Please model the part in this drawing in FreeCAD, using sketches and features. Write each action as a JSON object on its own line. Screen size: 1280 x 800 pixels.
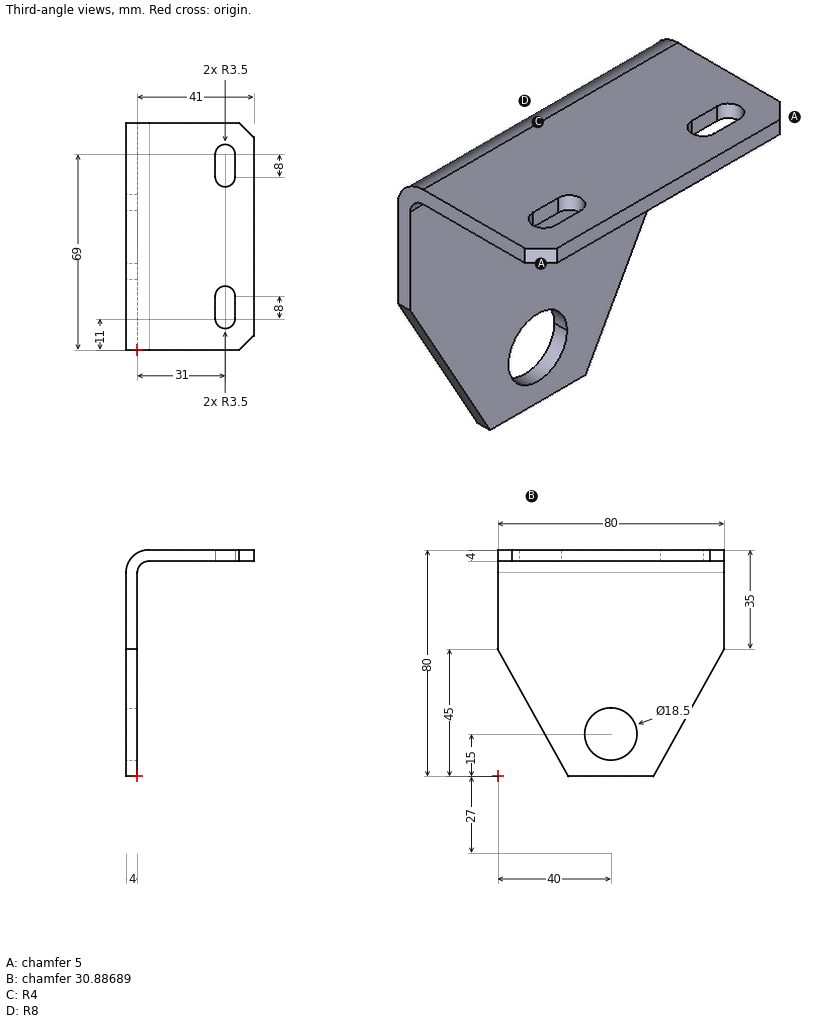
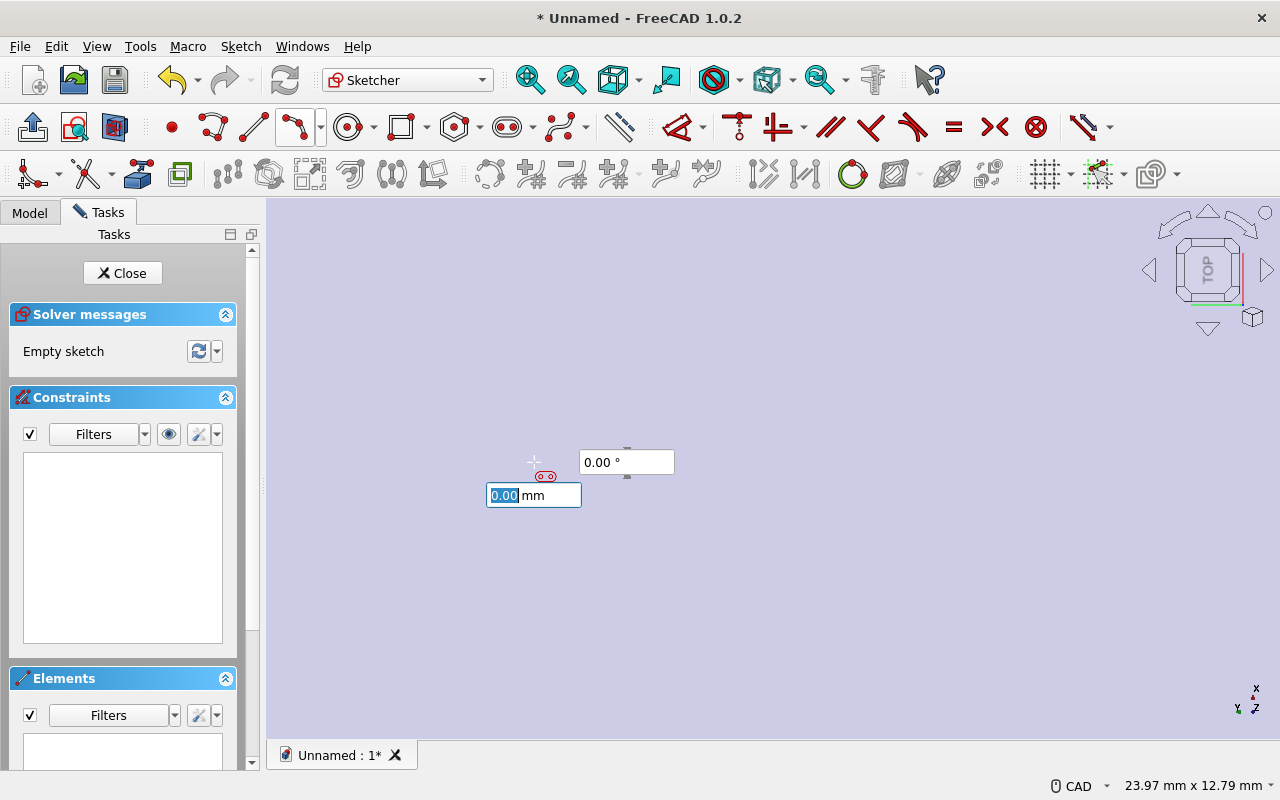
{"action": "left_click", "coordinate": [873, 462]}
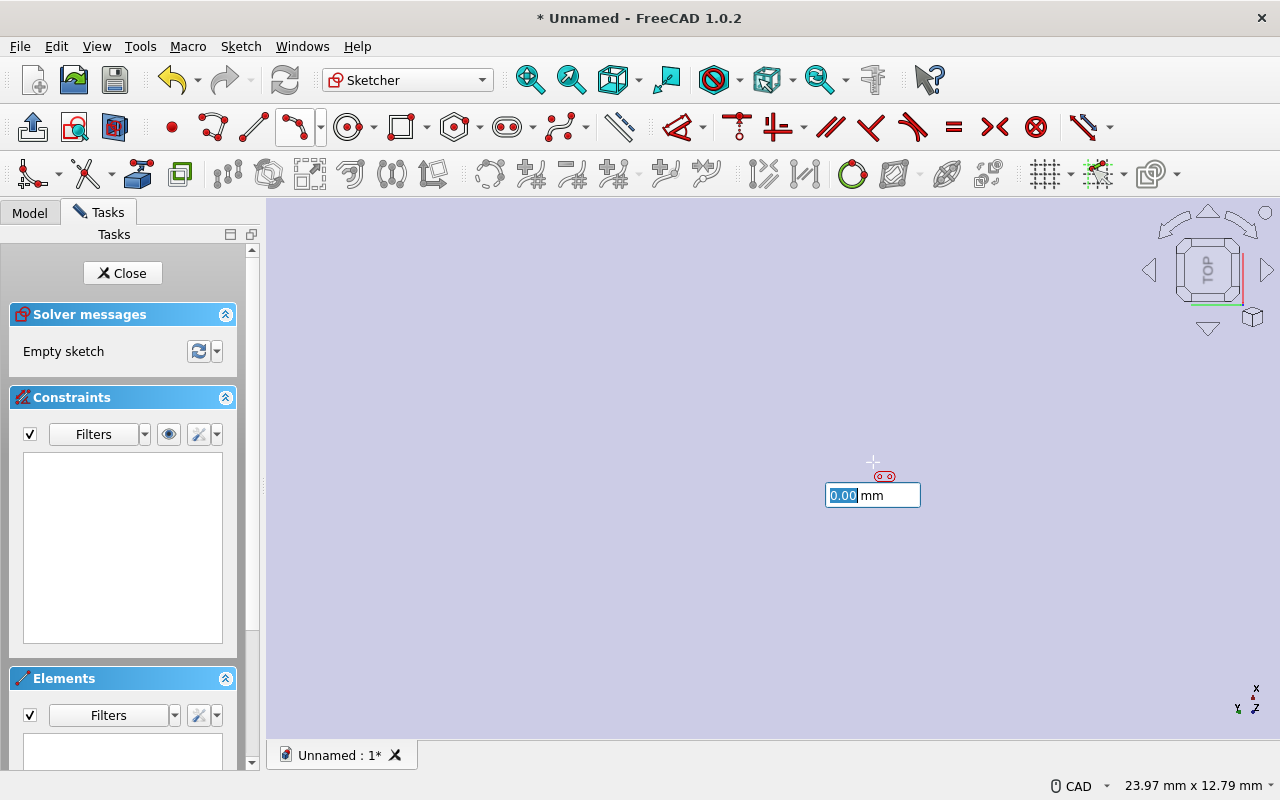
{"action": "left_click", "coordinate": [704, 314]}
{"action": "key", "text": "Escape"}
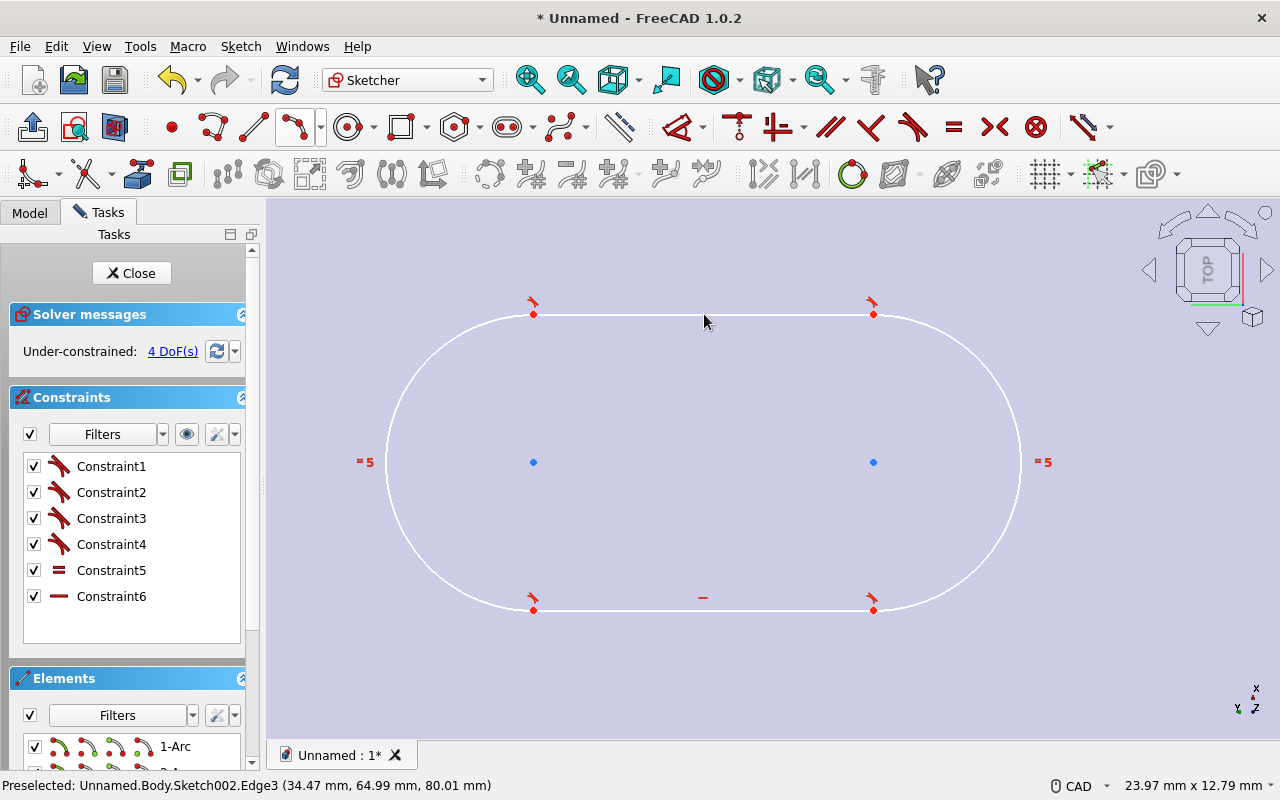
{"action": "left_click", "coordinate": [676, 128]}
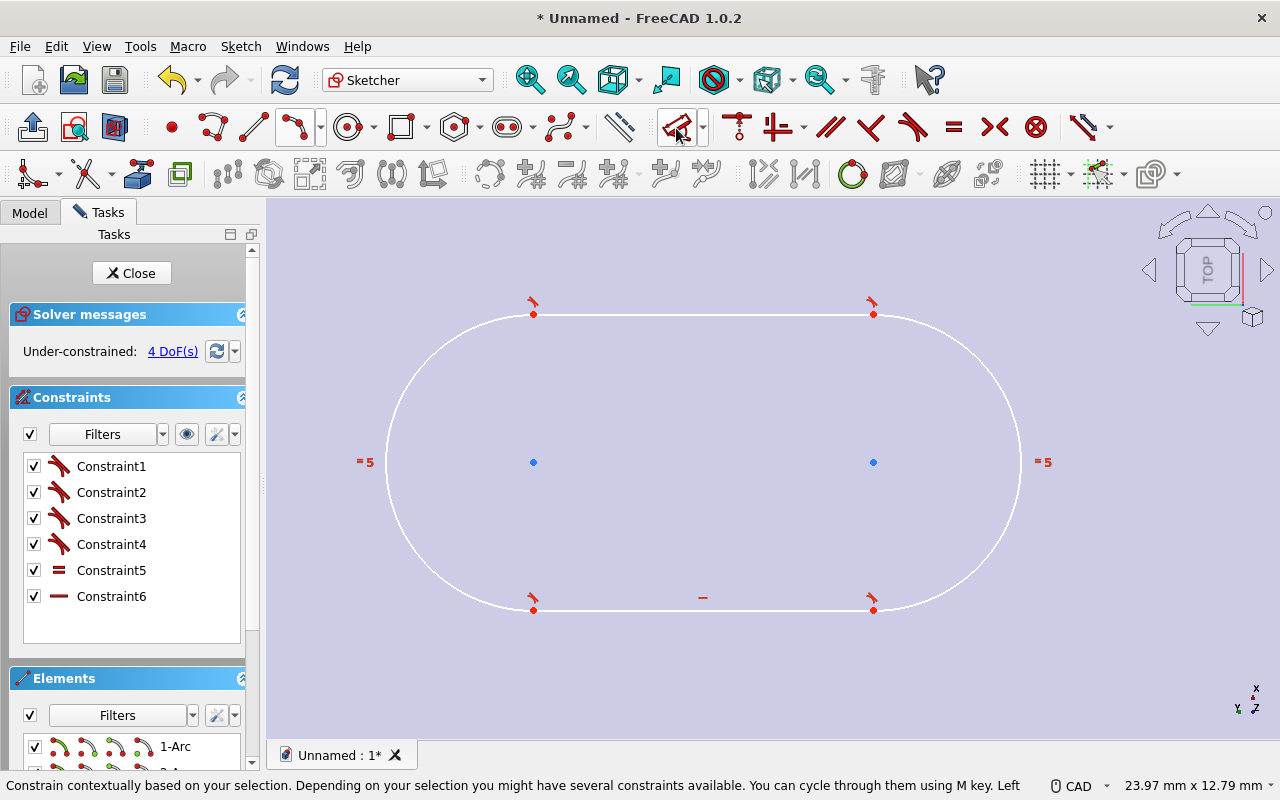
{"action": "left_click", "coordinate": [414, 376]}
{"action": "left_click", "coordinate": [388, 357]}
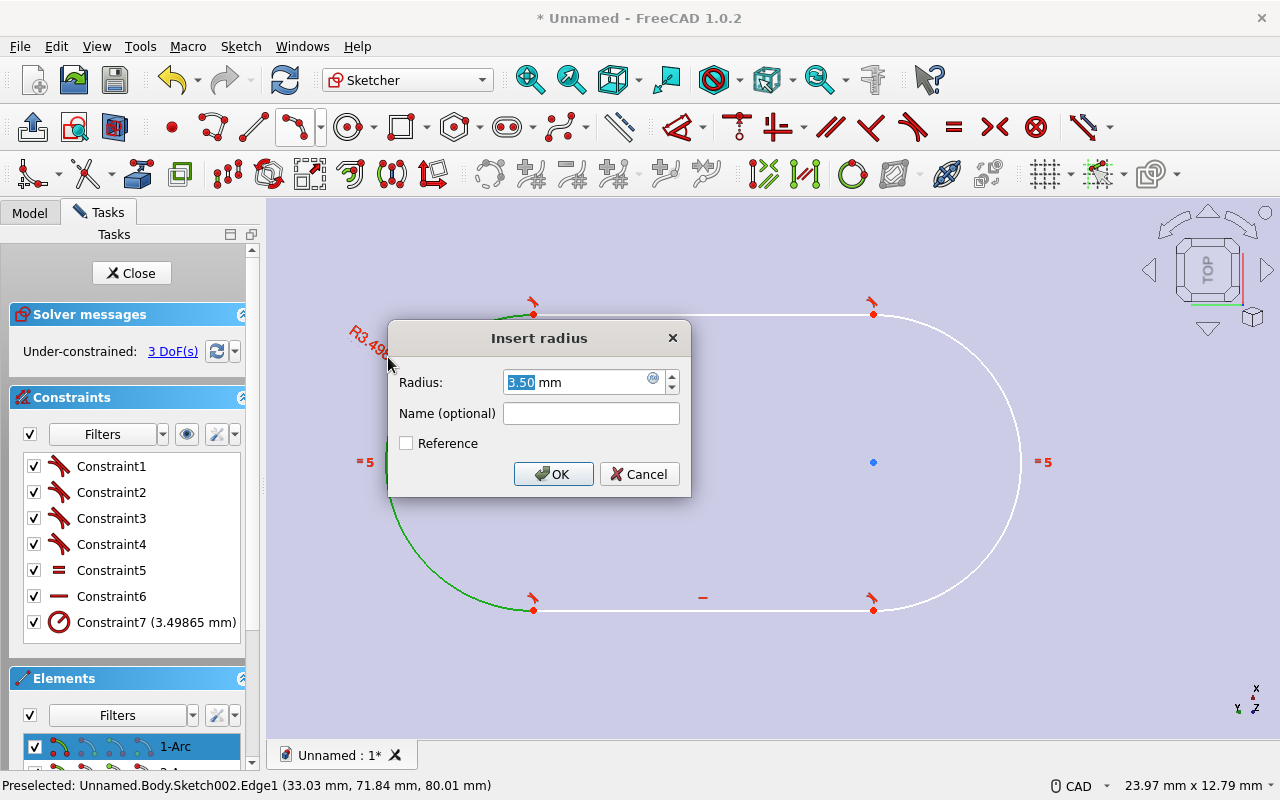
{"action": "type", "text": "3.5"}
{"action": "key", "text": "Return"}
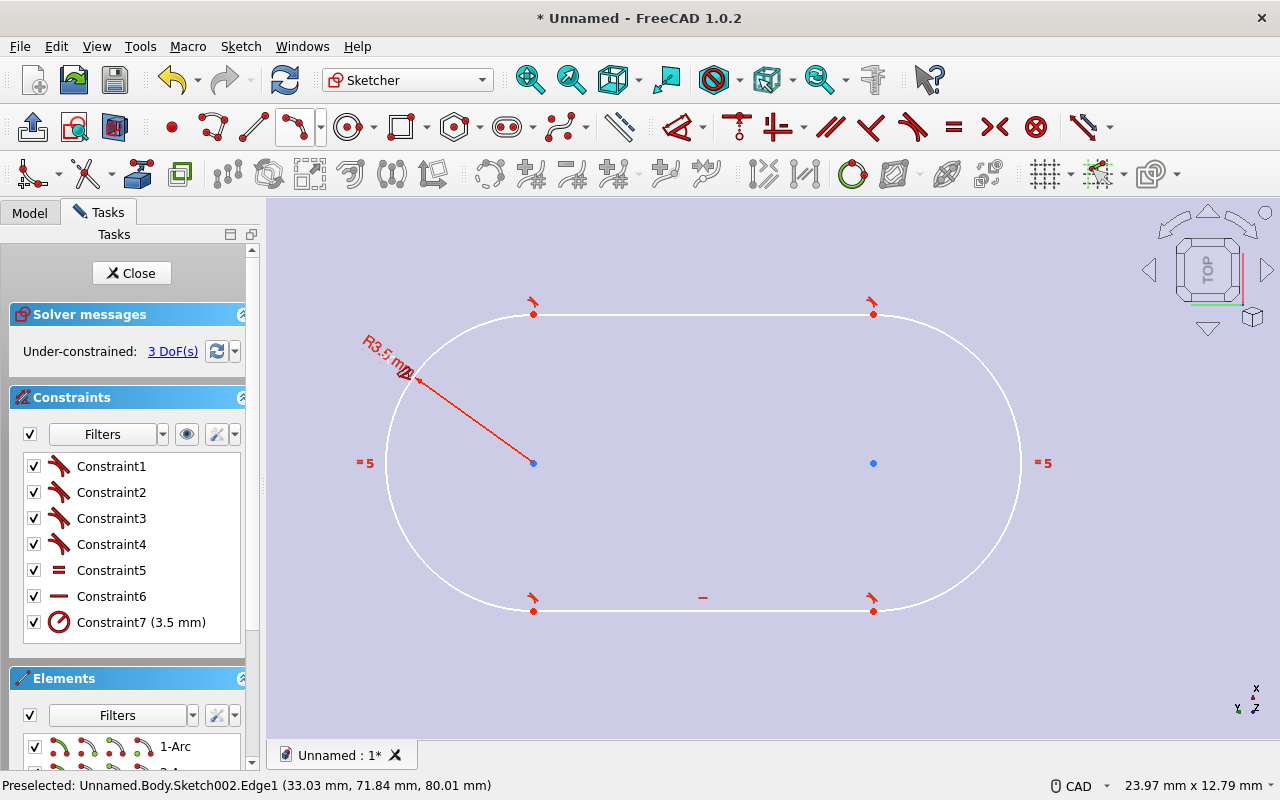
{"action": "left_click", "coordinate": [636, 315]}
{"action": "left_click", "coordinate": [703, 281]}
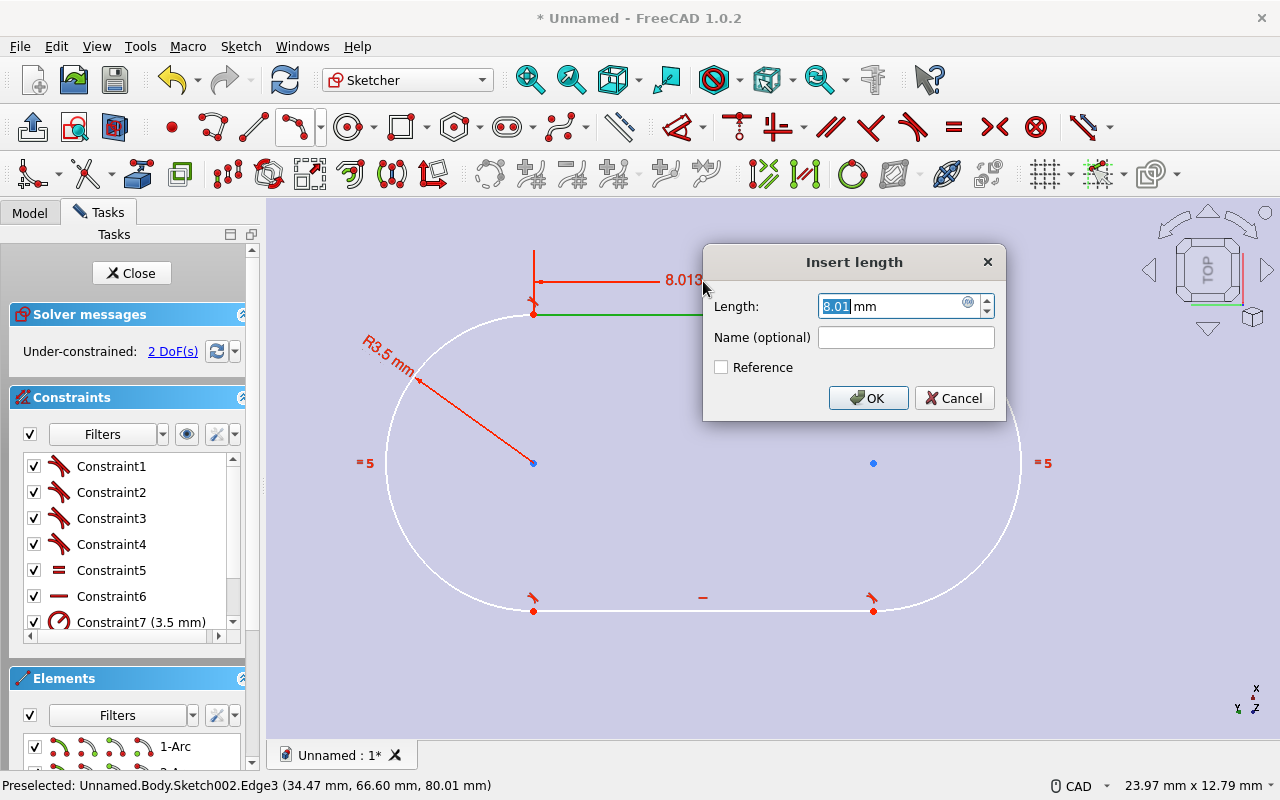
{"action": "type", "text": "8"}
{"action": "key", "text": "Return"}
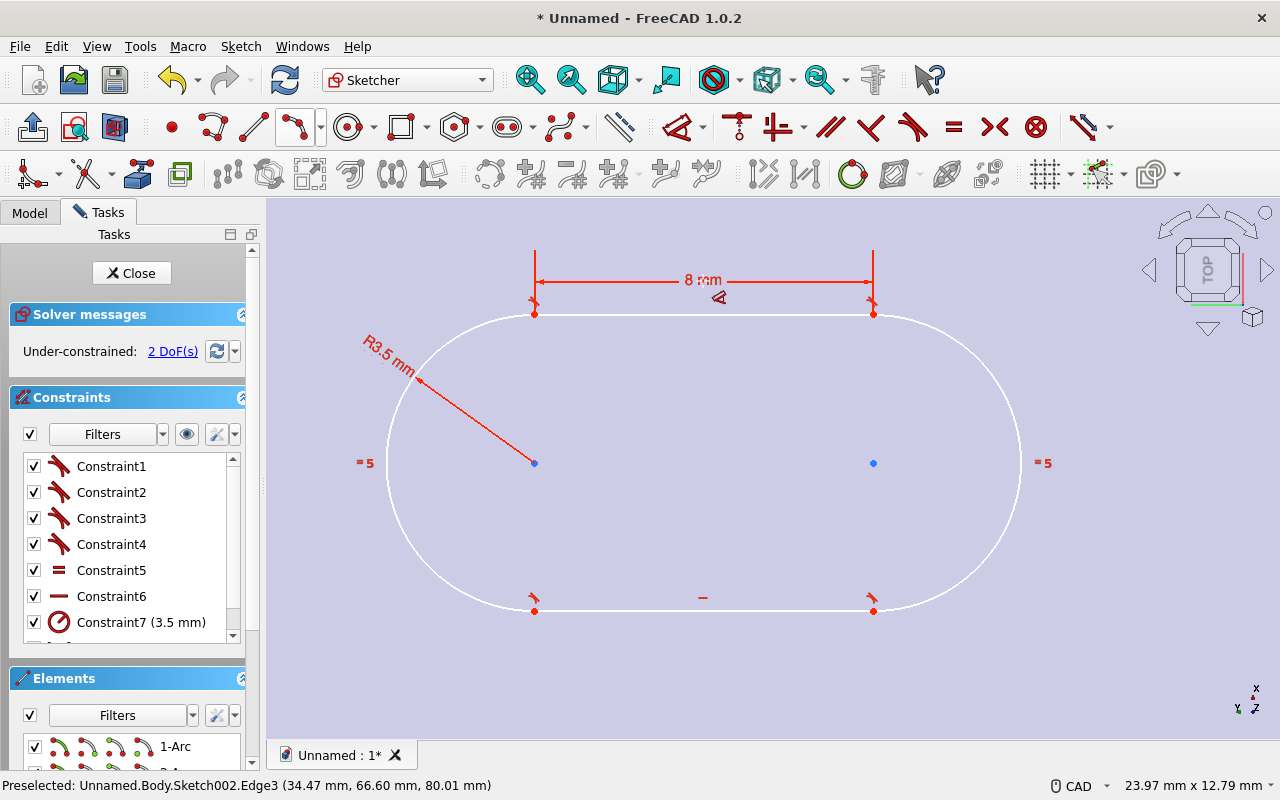
{"action": "left_click", "coordinate": [535, 315]}
{"action": "left_click", "coordinate": [825, 281]}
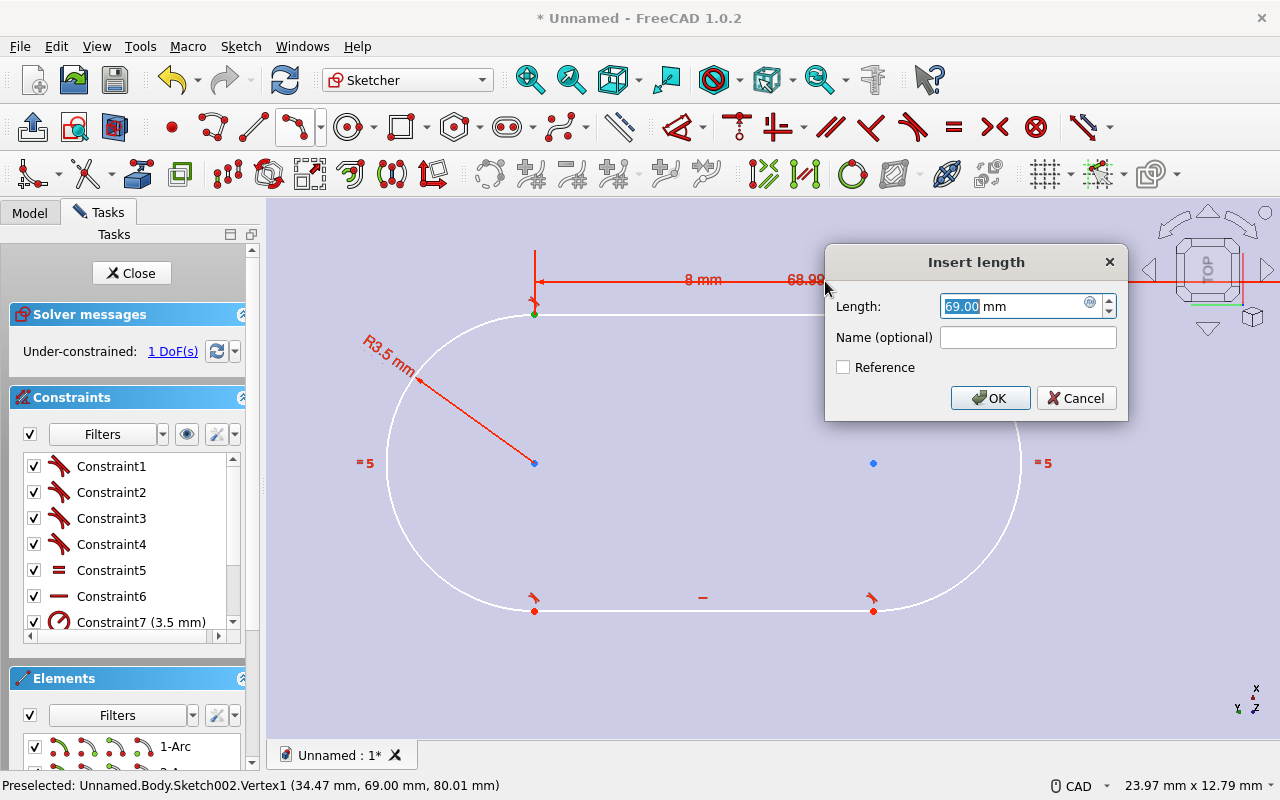
{"action": "type", "text": "69"}
{"action": "key", "text": "Return"}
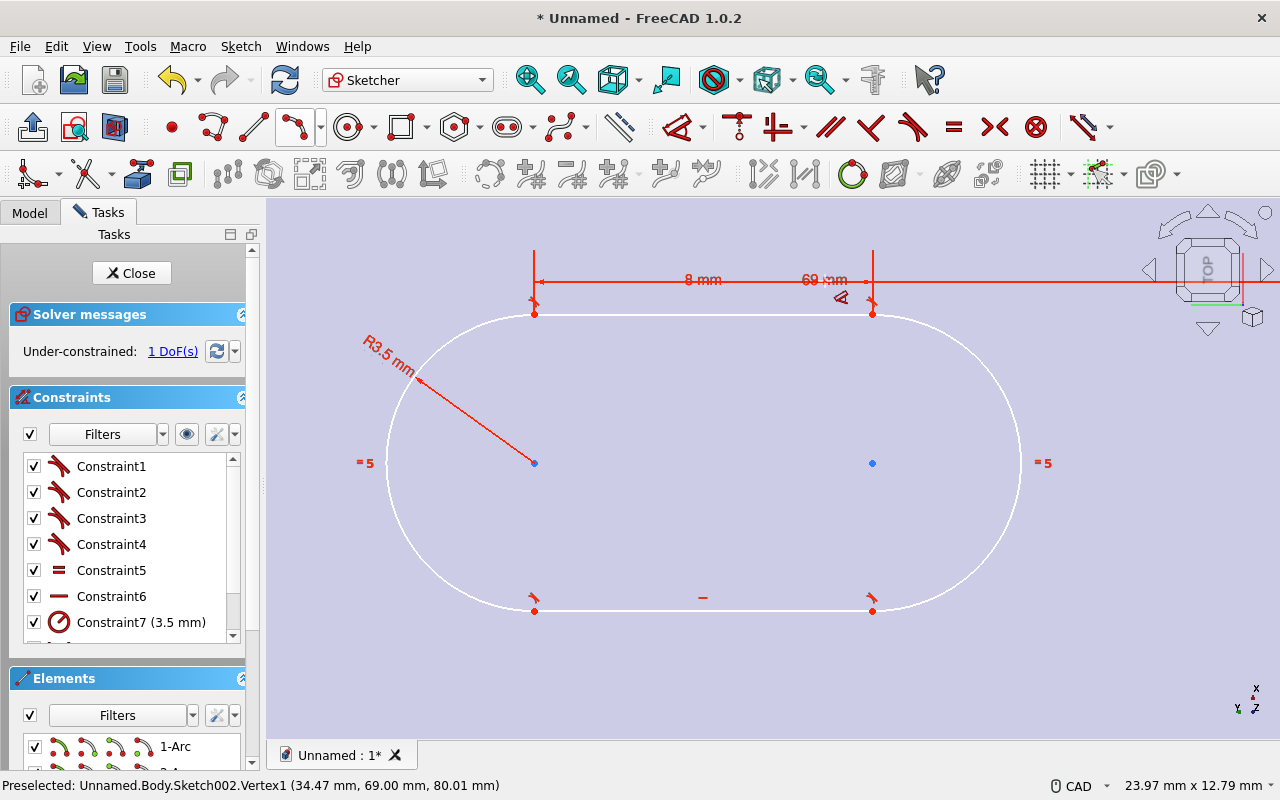
{"action": "left_click", "coordinate": [534, 463]}
{"action": "left_click", "coordinate": [500, 587]}